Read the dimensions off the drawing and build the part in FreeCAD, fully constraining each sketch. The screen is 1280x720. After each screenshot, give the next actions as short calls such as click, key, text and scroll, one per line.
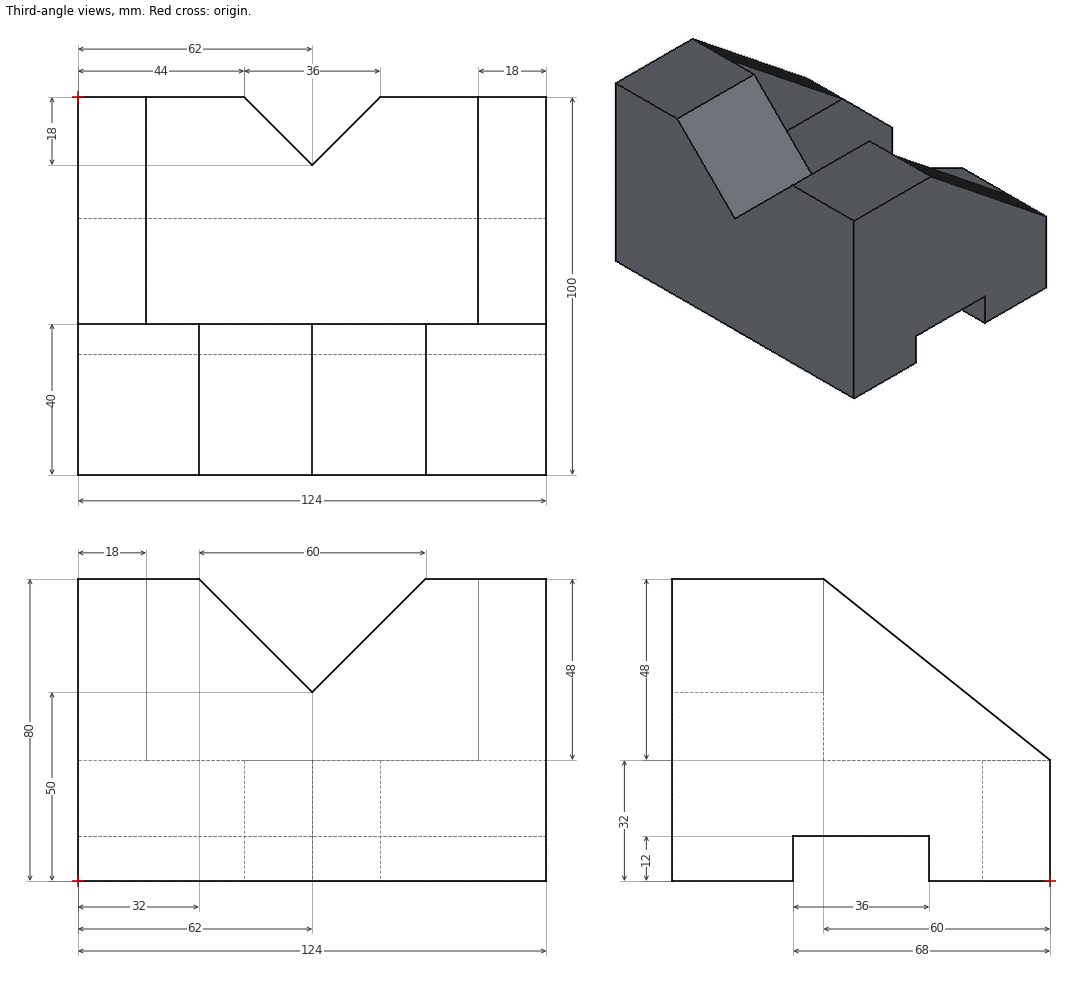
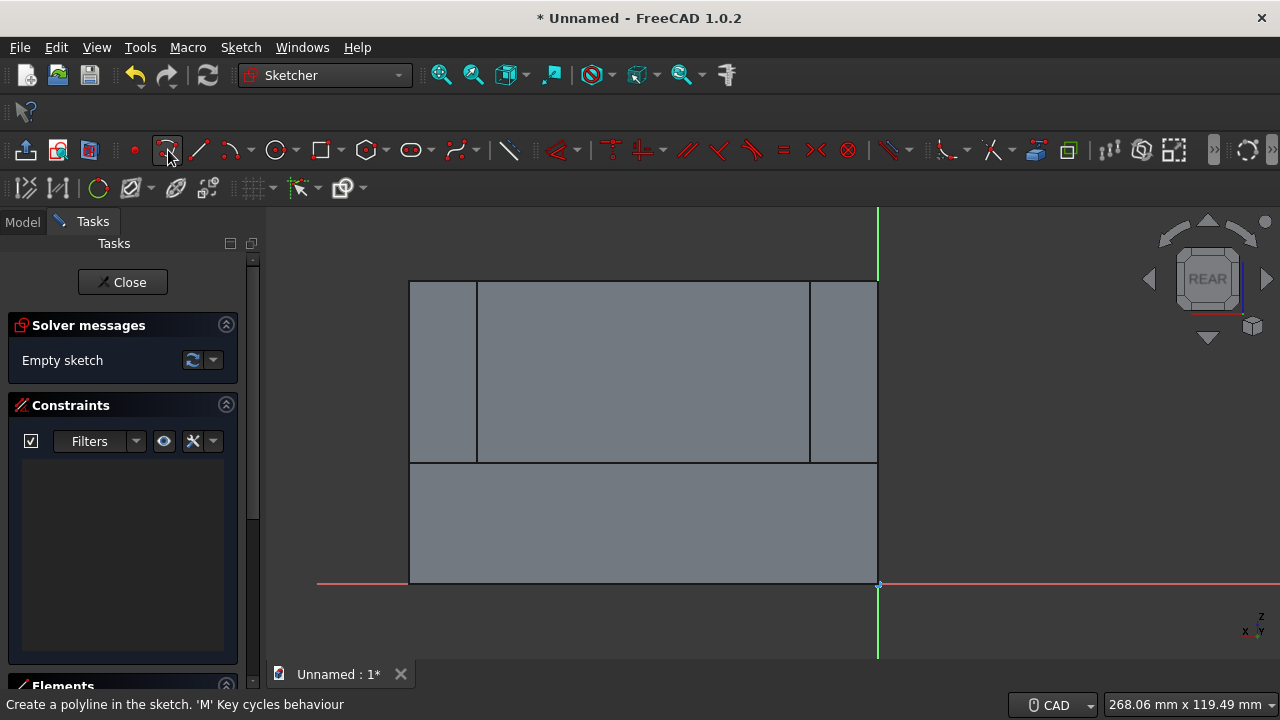
click(644, 395)
click(757, 281)
click(530, 281)
click(644, 396)
key(Escape)
key(Escape)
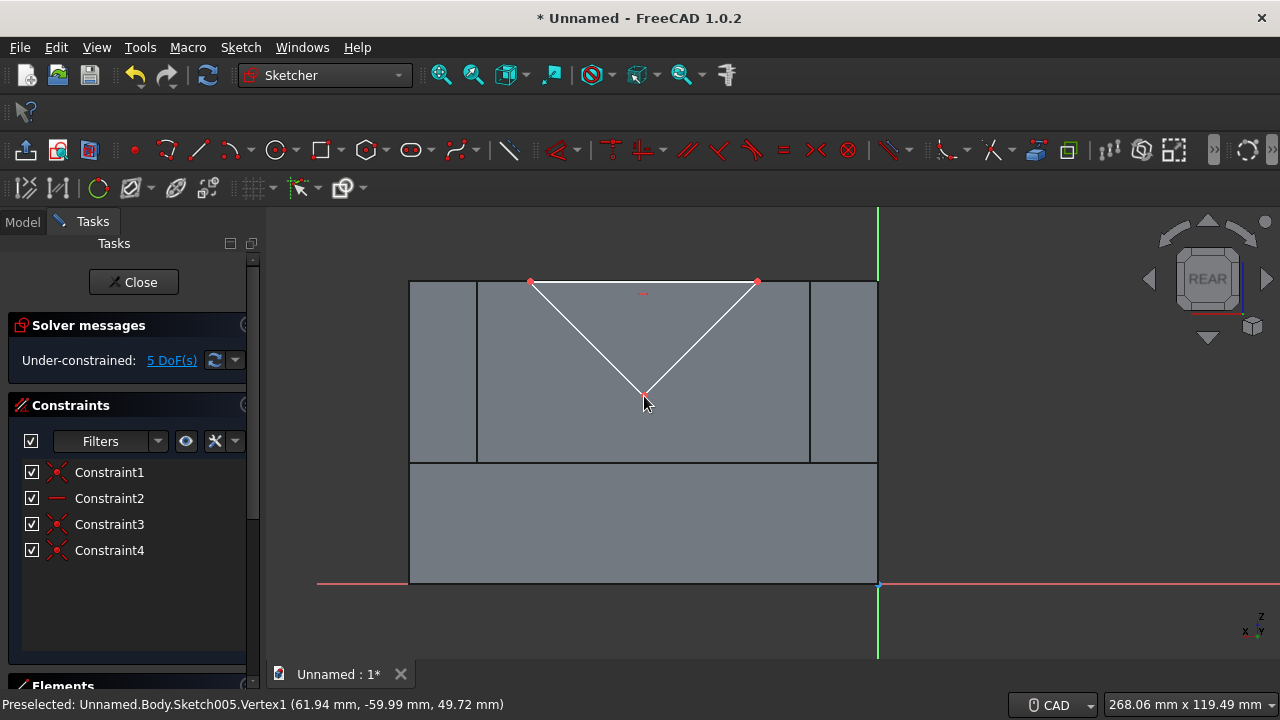
click(556, 150)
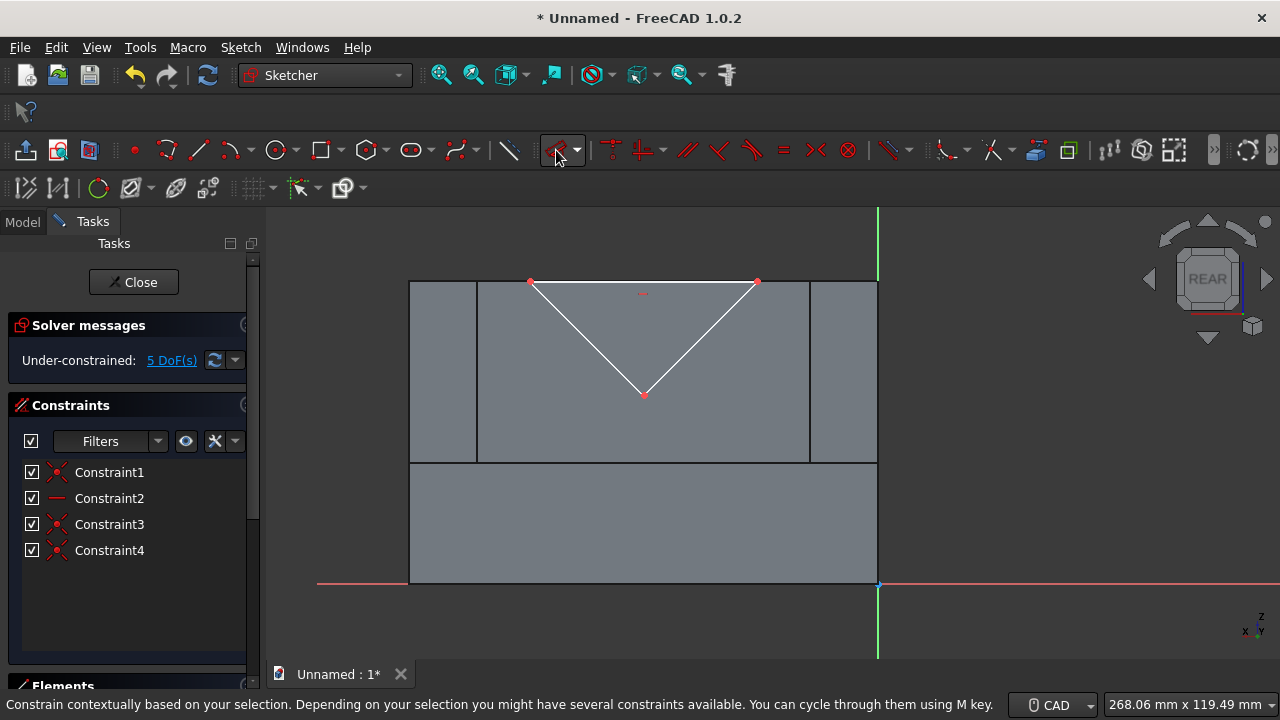
click(689, 282)
click(643, 248)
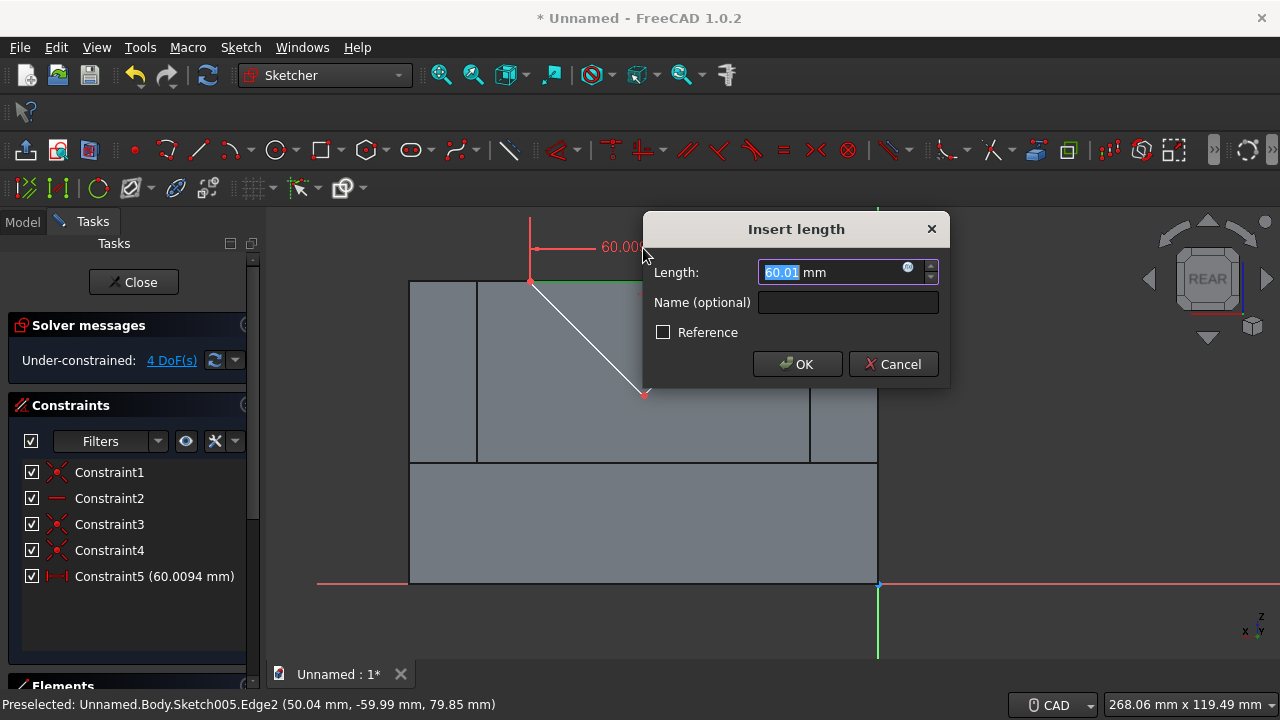
text(60)
key(Return)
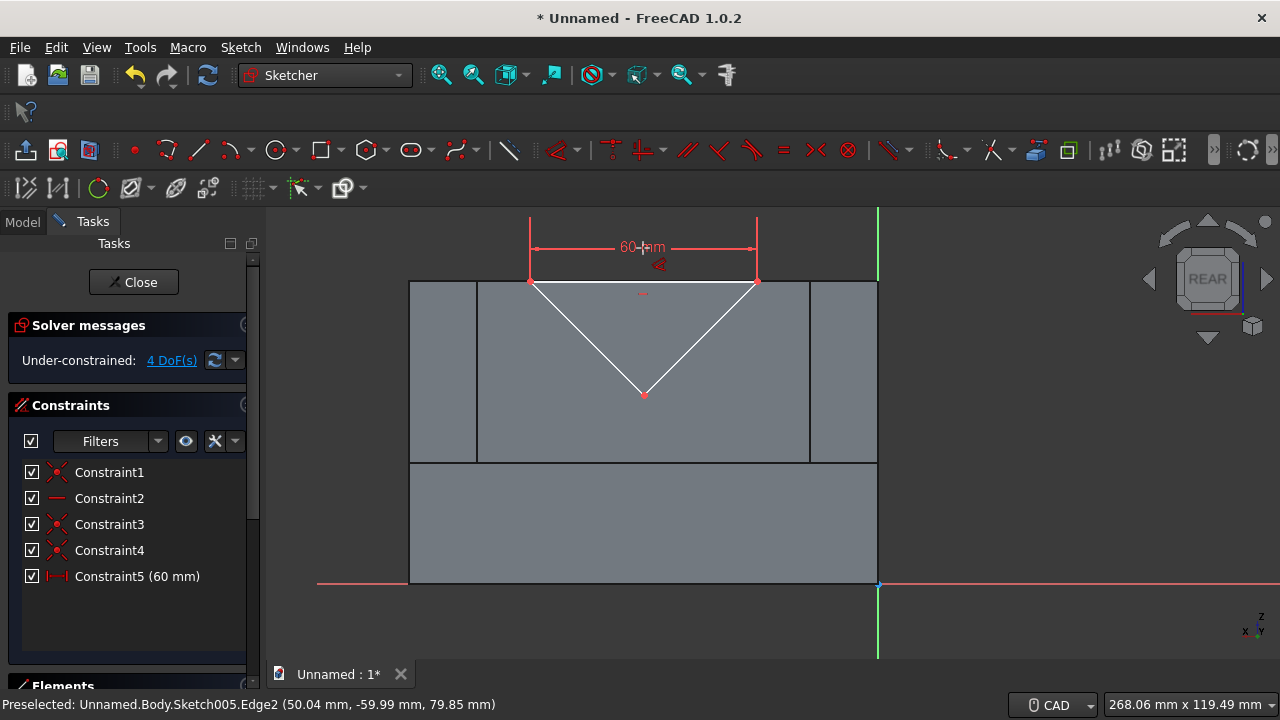
click(644, 396)
click(761, 618)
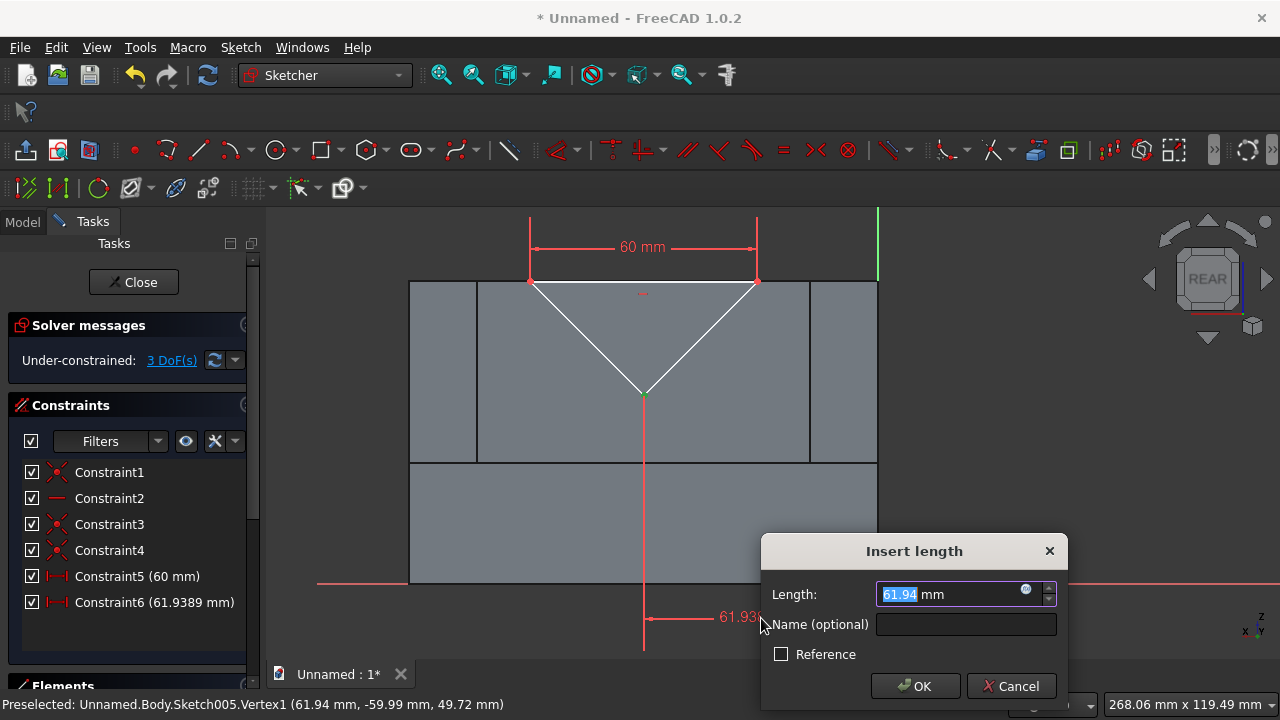
text(62)
key(Return)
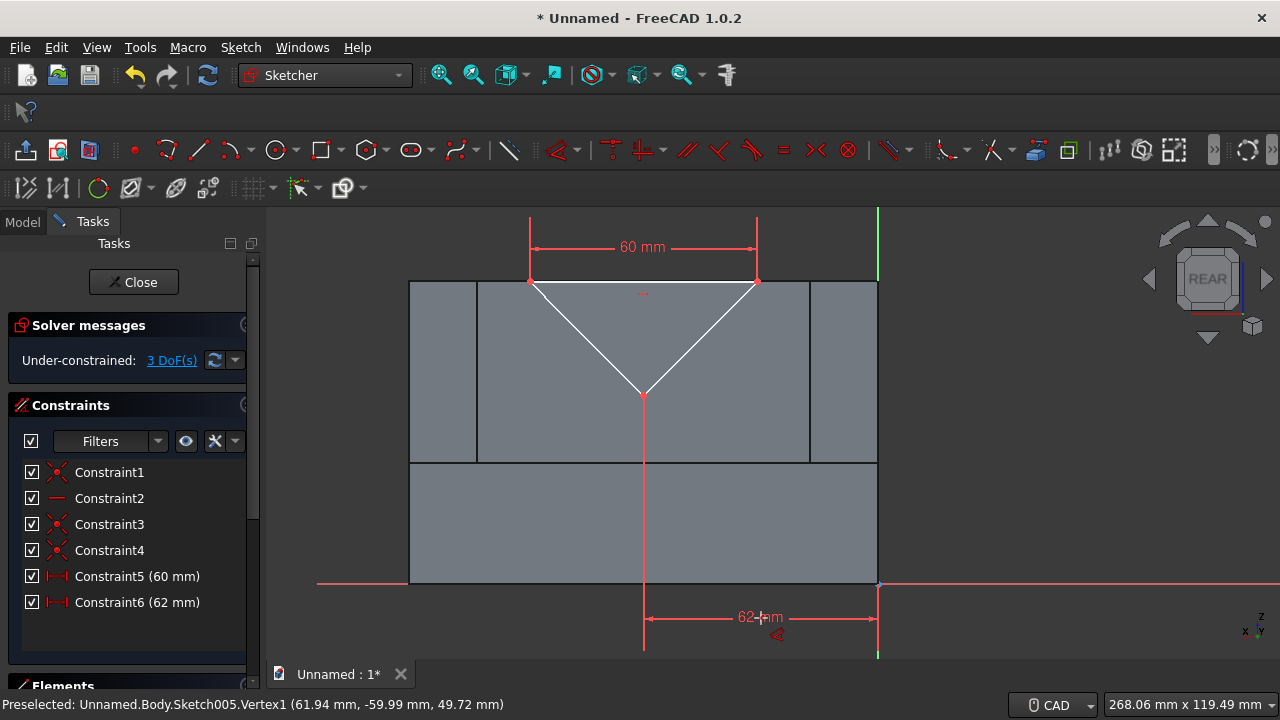
click(644, 396)
click(912, 490)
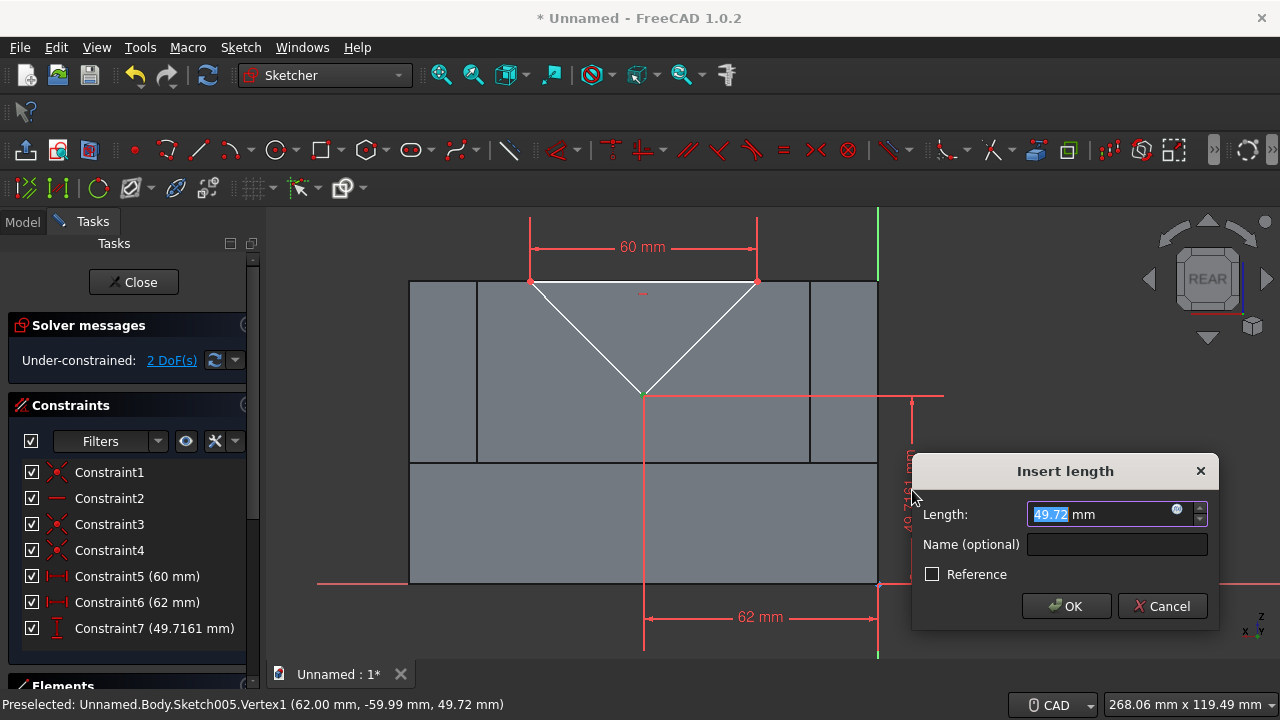
text(50)
key(Return)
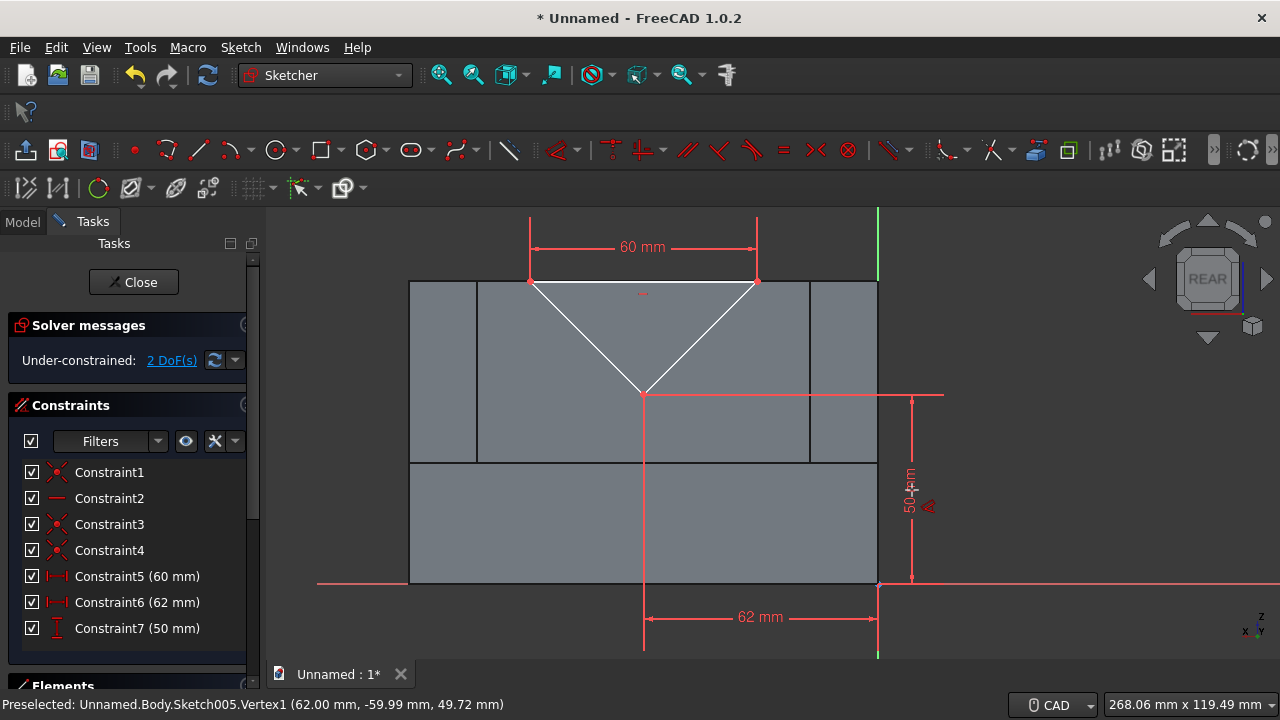
click(757, 282)
click(846, 618)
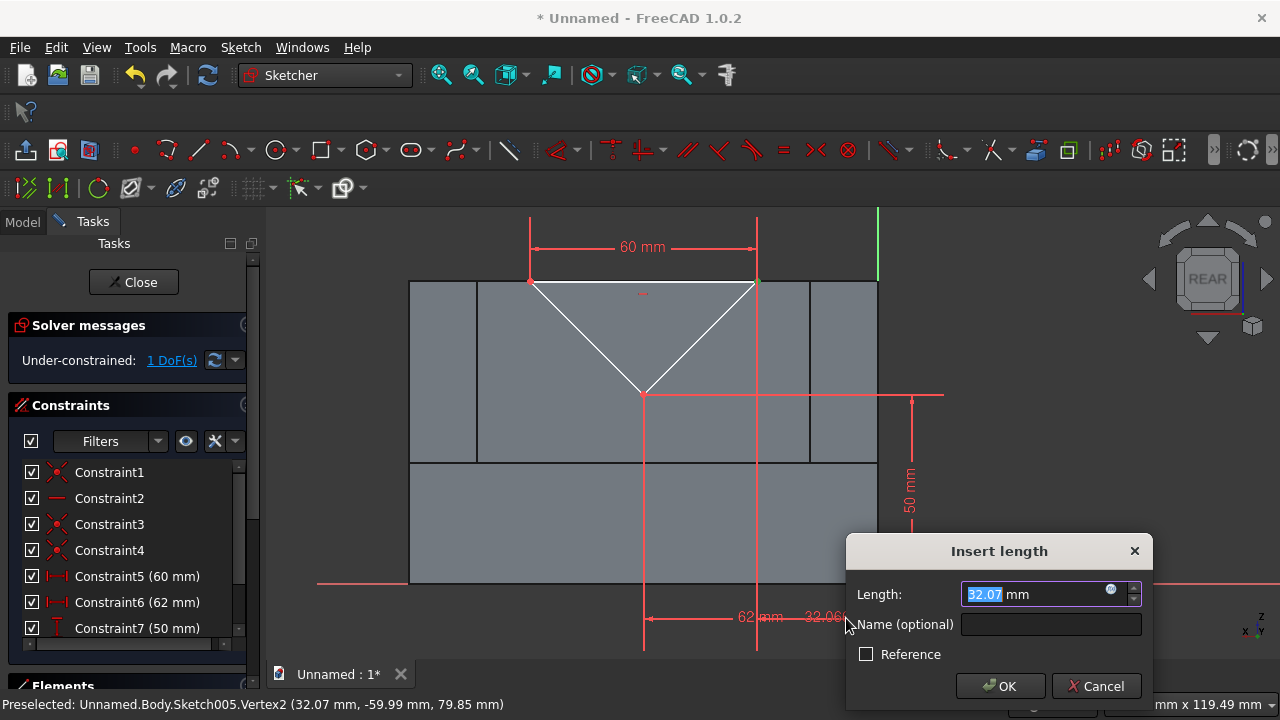
text(32)
key(Return)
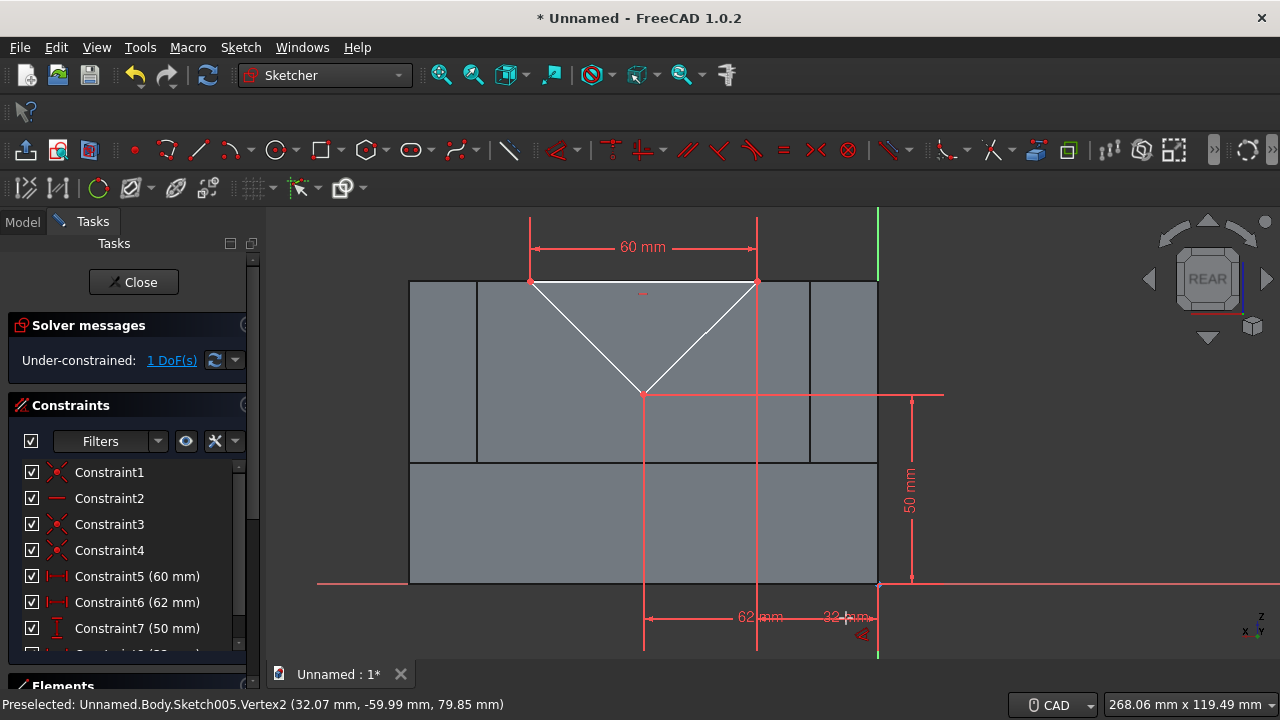
click(757, 282)
click(912, 433)